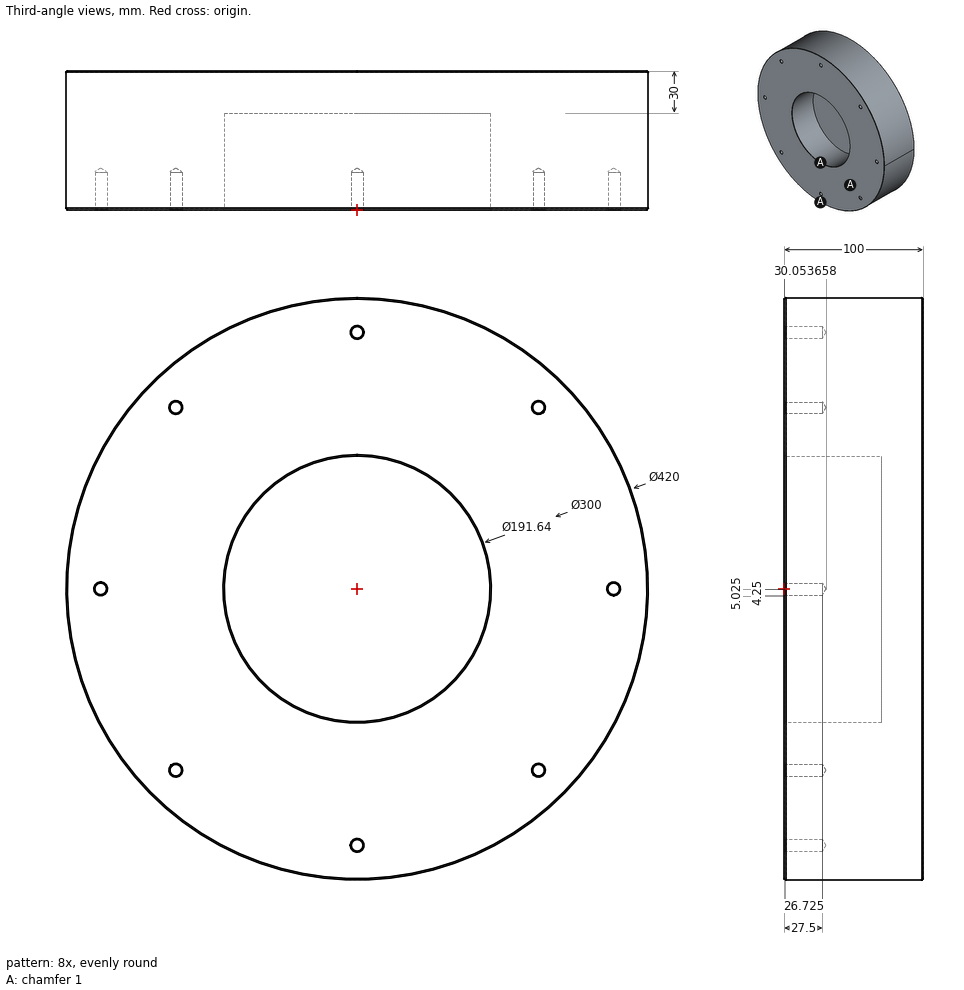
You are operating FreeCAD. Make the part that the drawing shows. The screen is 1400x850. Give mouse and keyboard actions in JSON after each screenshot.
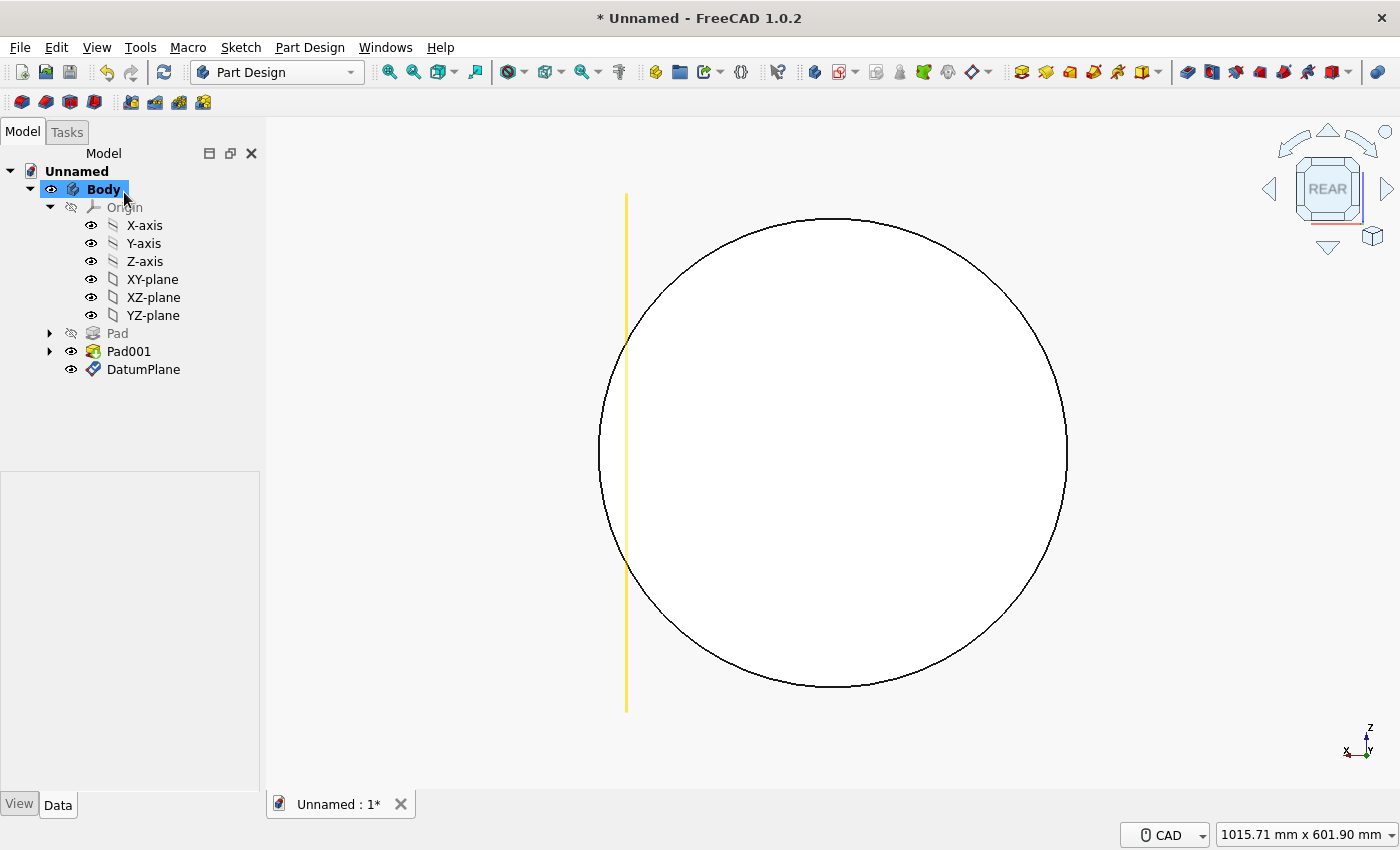
{"action": "left_click", "coordinate": [116, 369]}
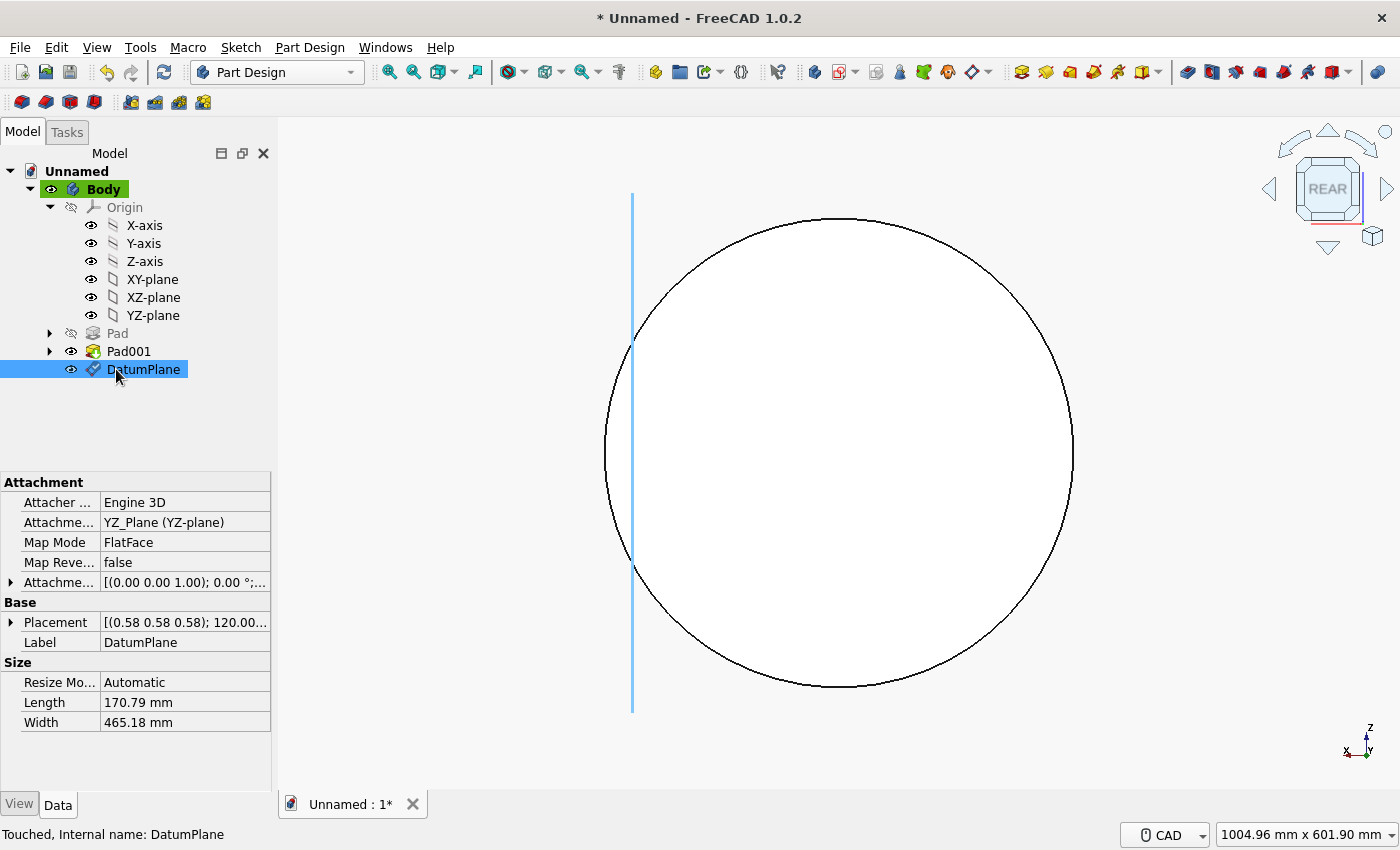
{"action": "left_click", "coordinate": [840, 72]}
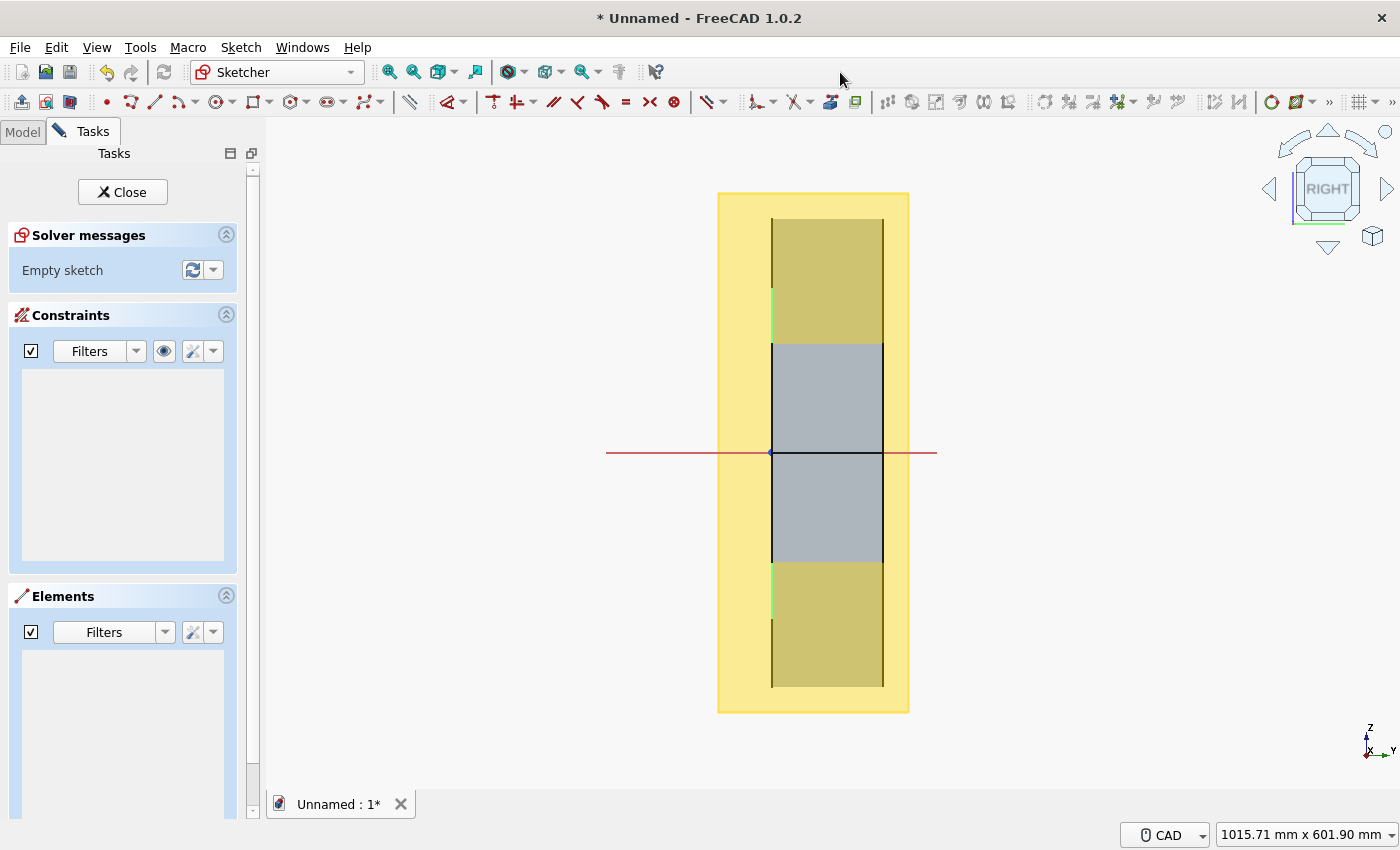
{"action": "key", "text": "q s"}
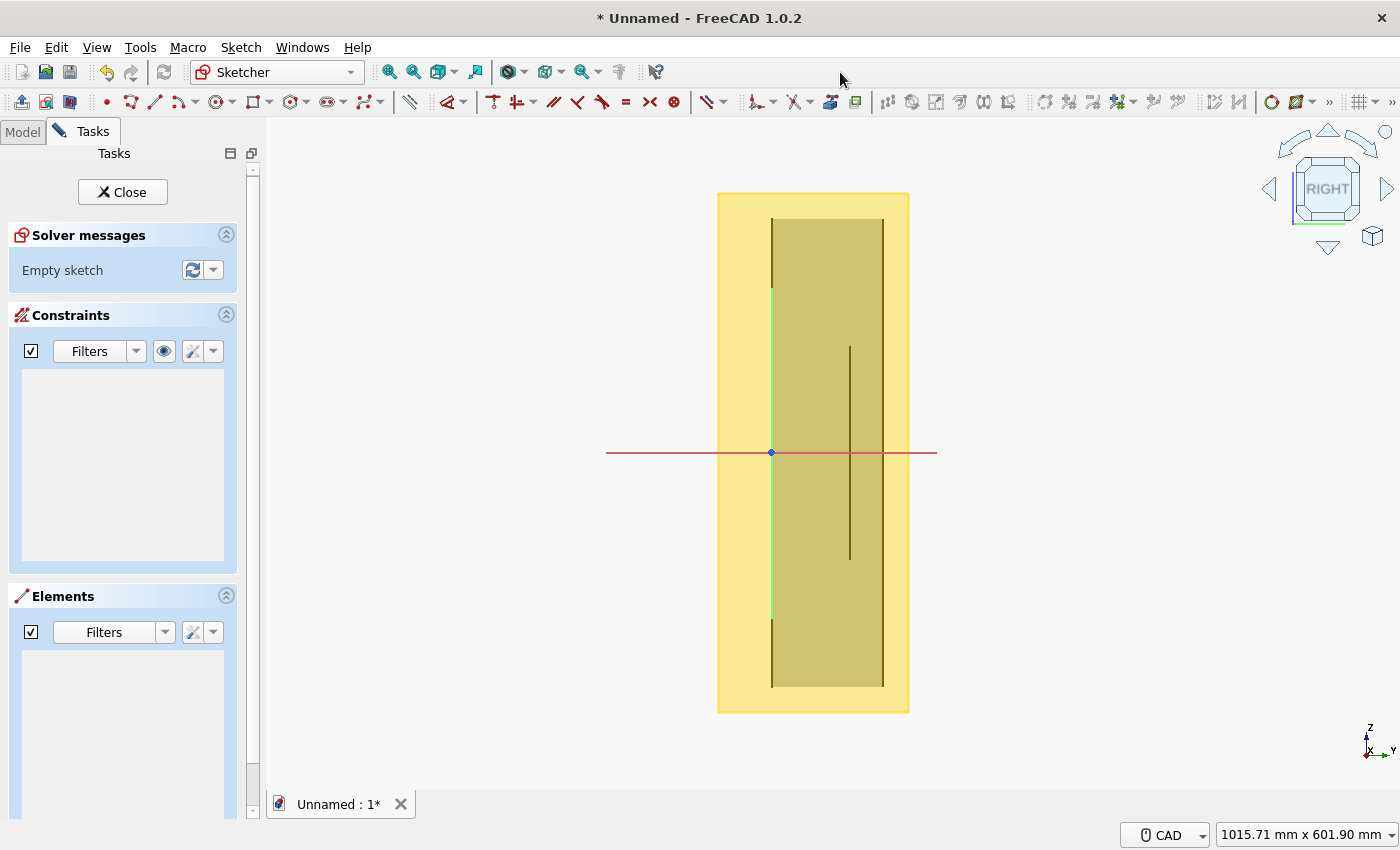
{"action": "scroll", "coordinate": [790, 456], "scroll_direction": "up", "scroll_amount": 15}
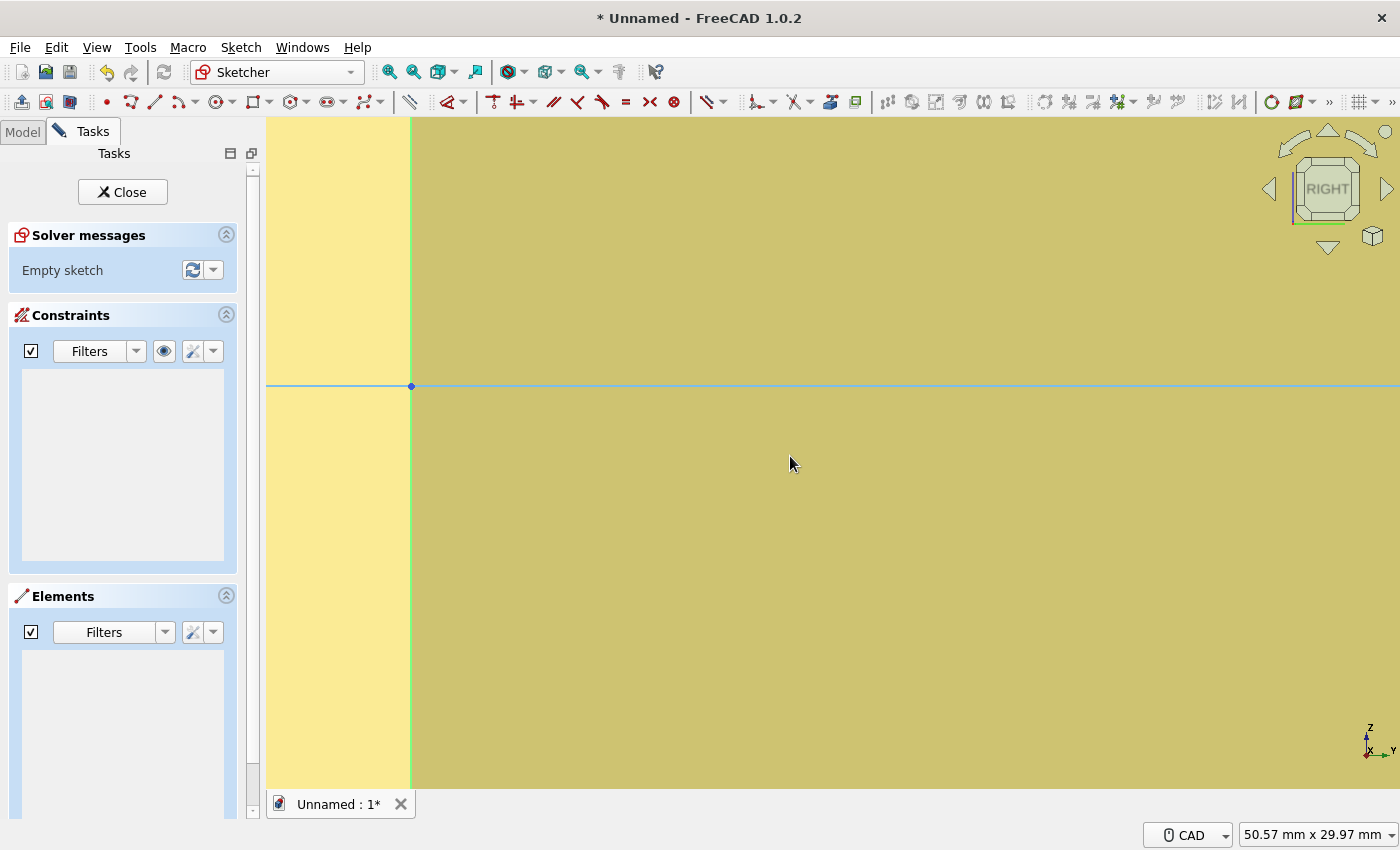
{"action": "key", "text": "g m"}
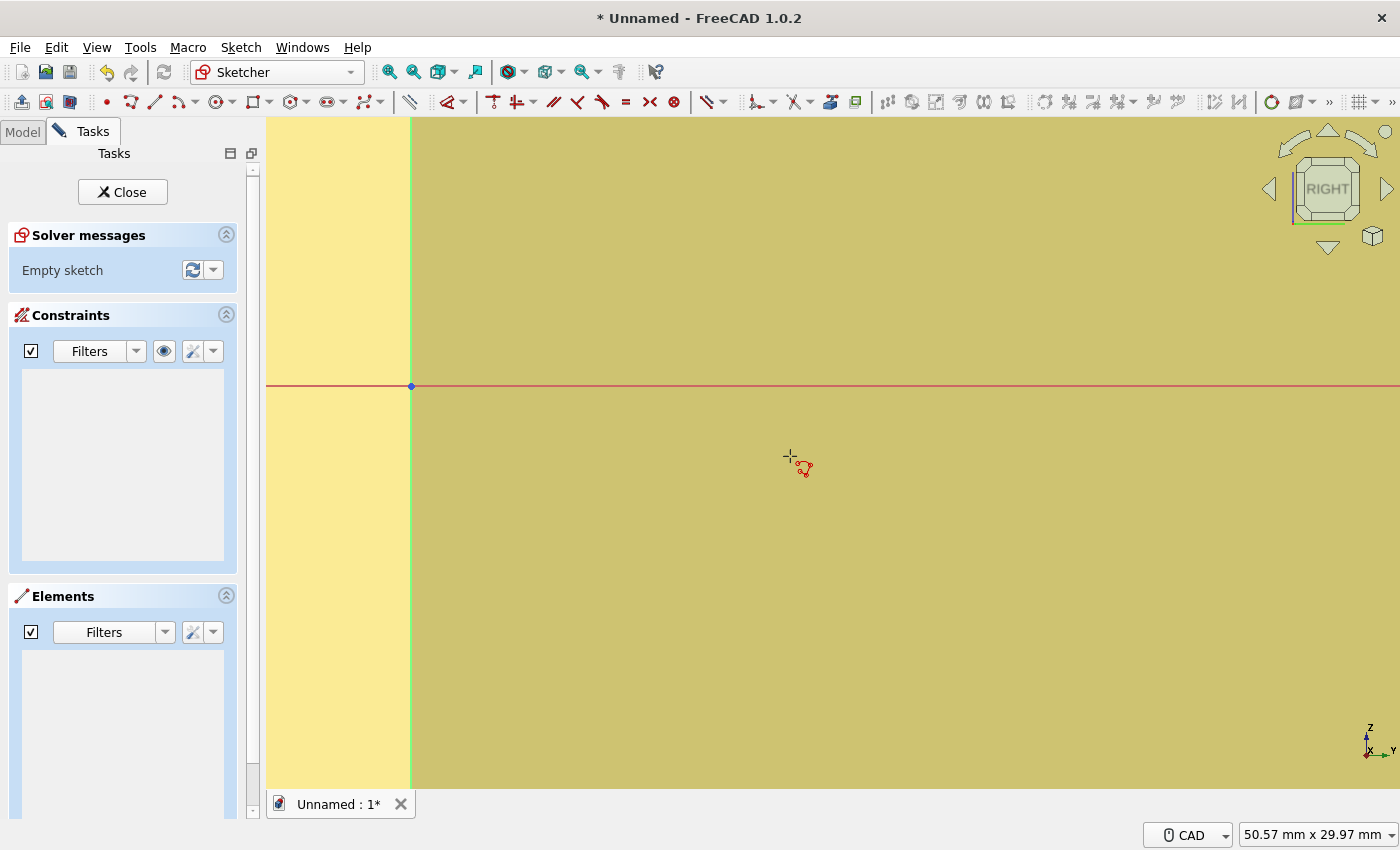
{"action": "left_click", "coordinate": [411, 386]}
{"action": "left_click", "coordinate": [420, 499]}
{"action": "left_click", "coordinate": [429, 481]}
{"action": "left_click", "coordinate": [1028, 481]}
{"action": "left_click", "coordinate": [1085, 395]}
{"action": "left_click", "coordinate": [411, 386]}
{"action": "key", "text": "Escape"}
{"action": "key", "text": "Escape"}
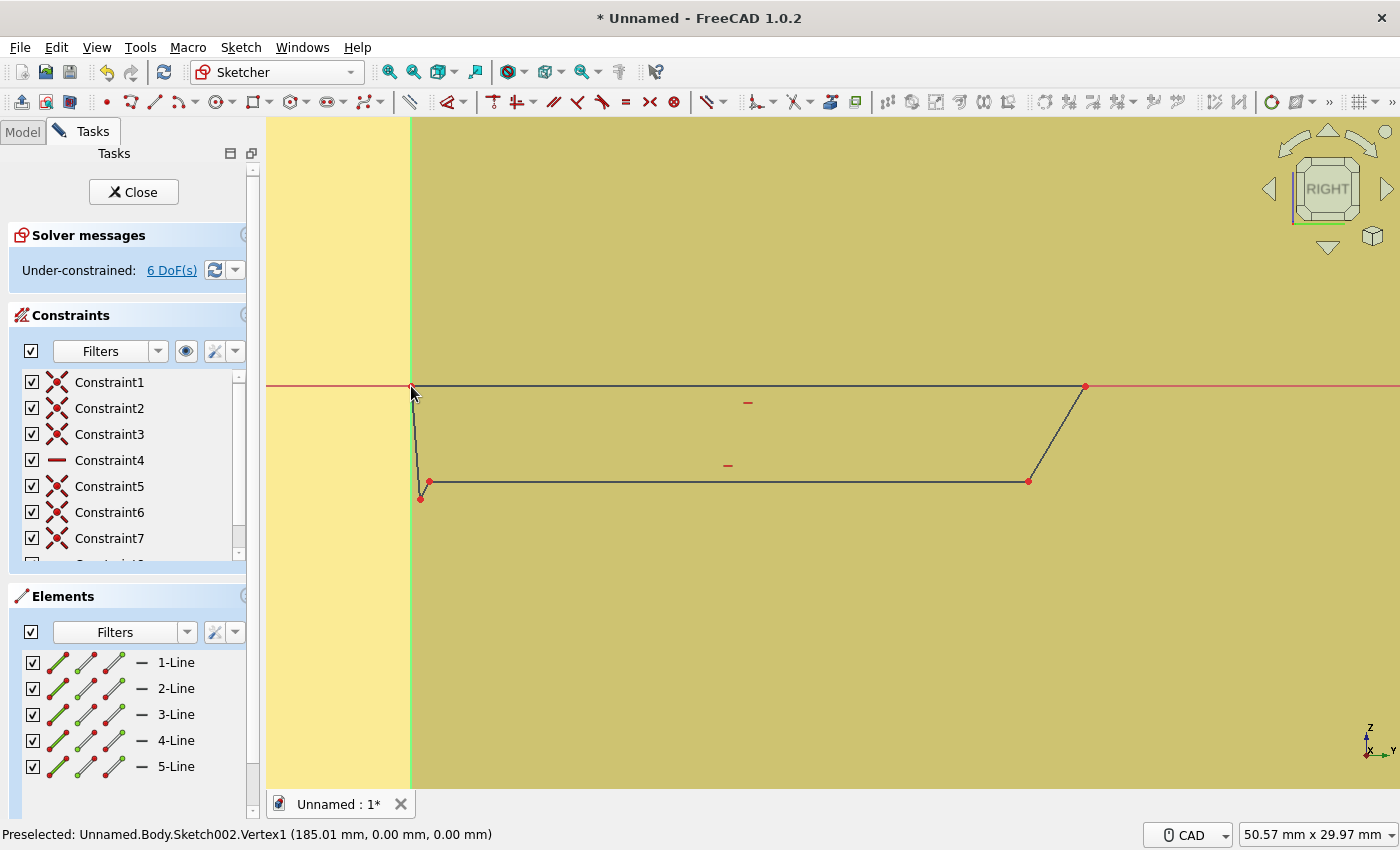
{"action": "left_click", "coordinate": [414, 420]}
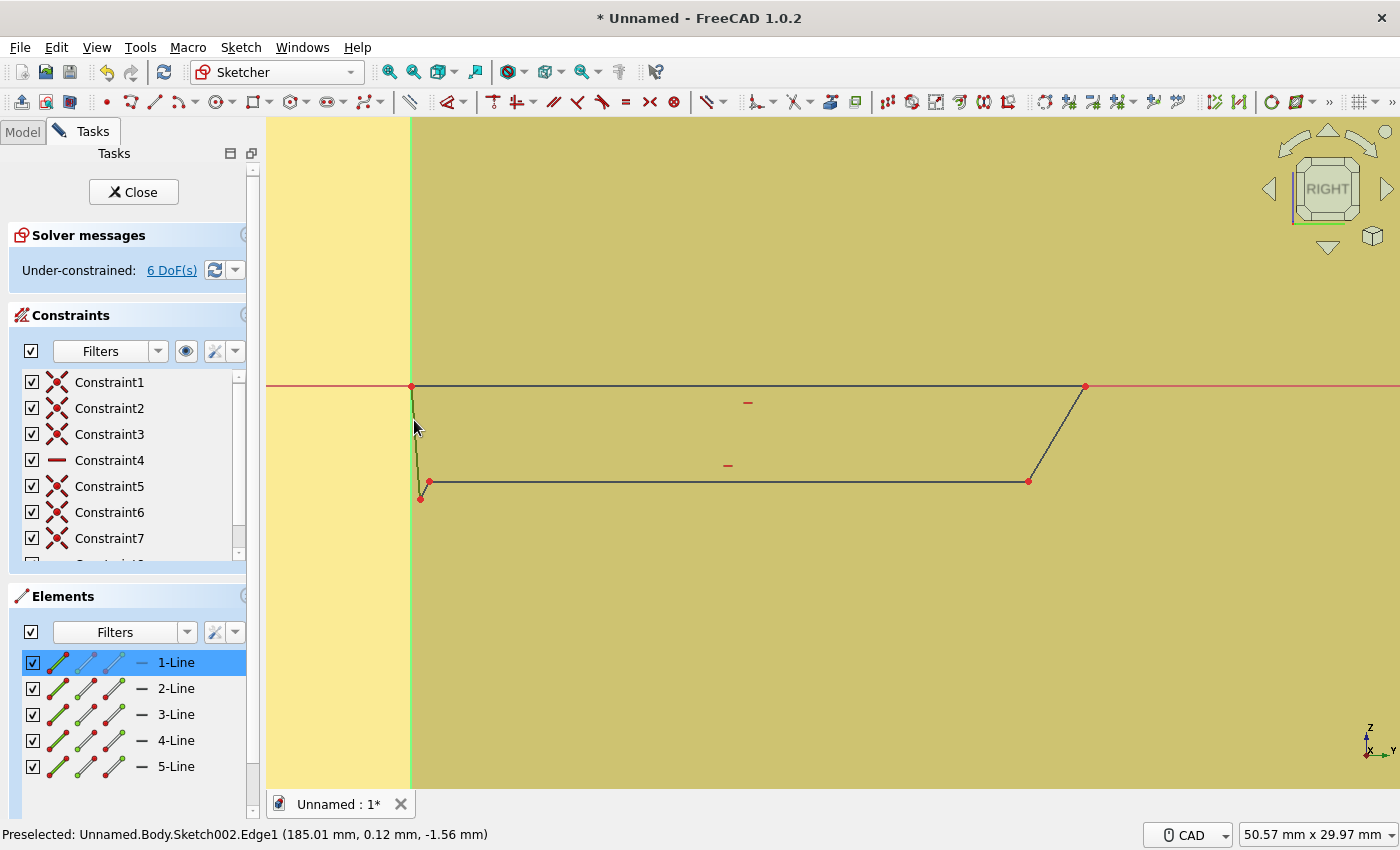
{"action": "key", "text": "v"}